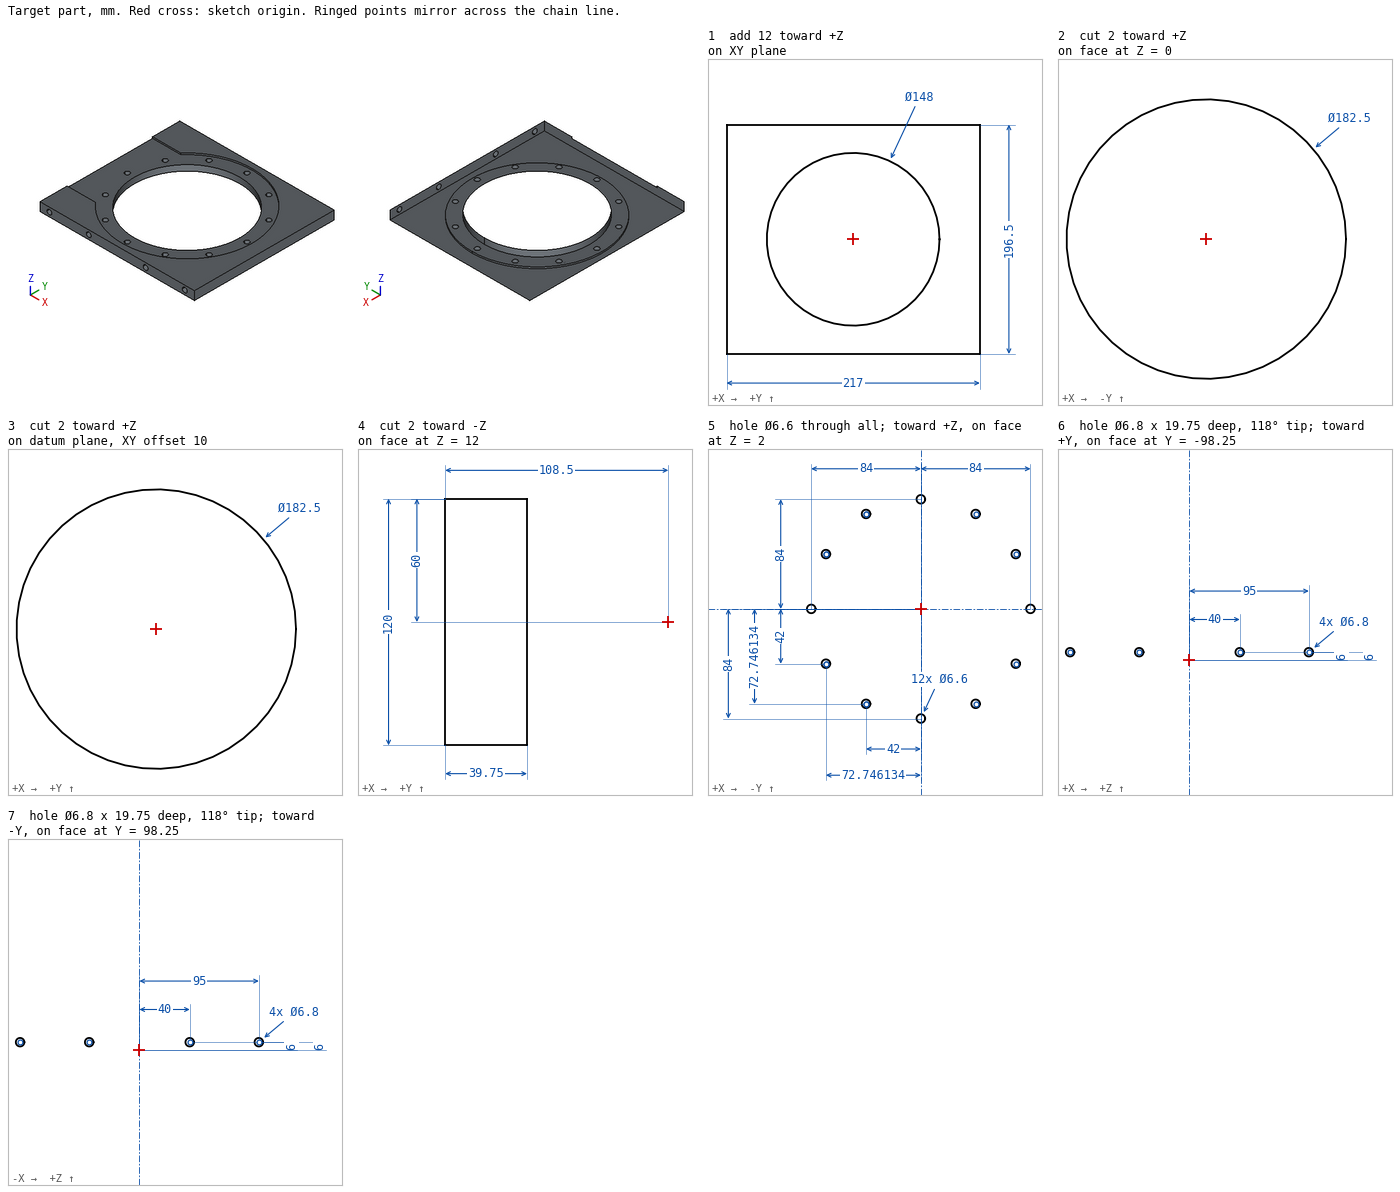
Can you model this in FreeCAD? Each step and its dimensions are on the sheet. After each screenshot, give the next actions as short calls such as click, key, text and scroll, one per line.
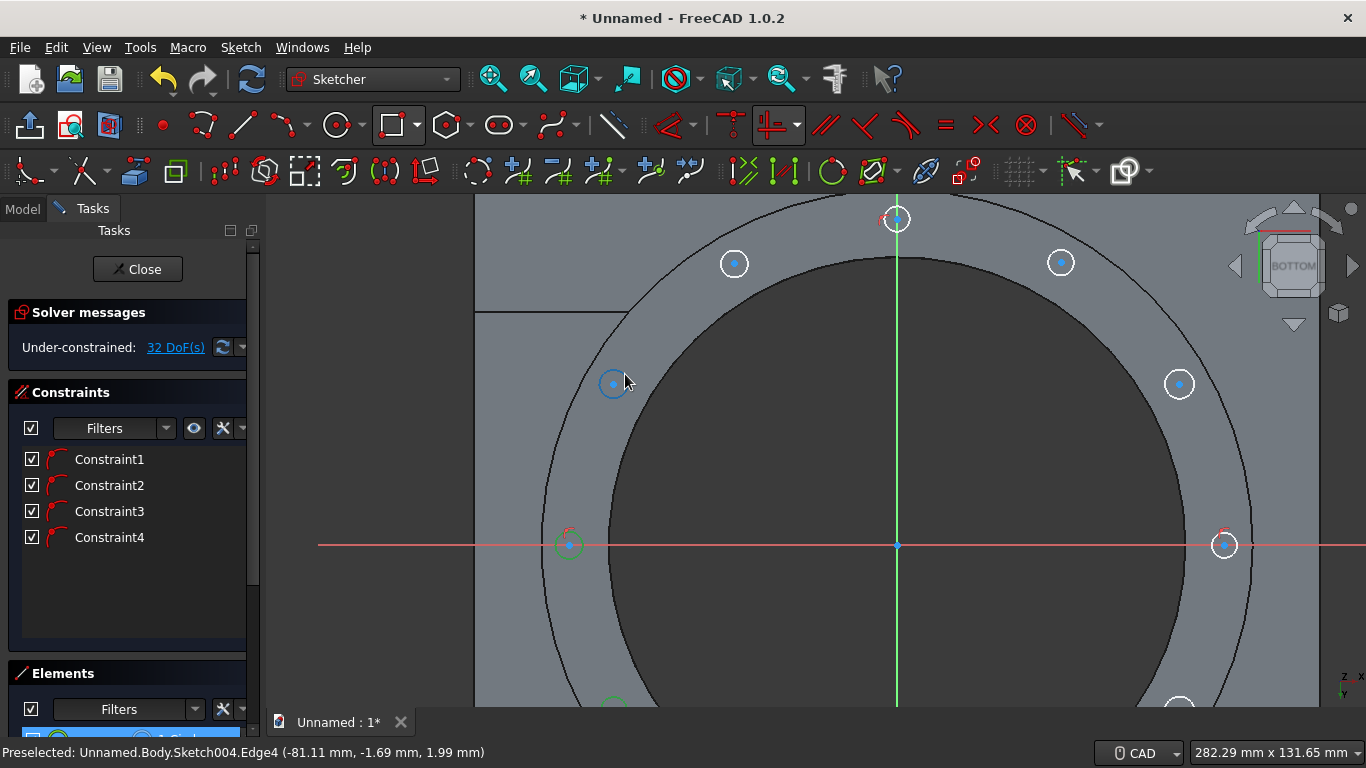
click(624, 374)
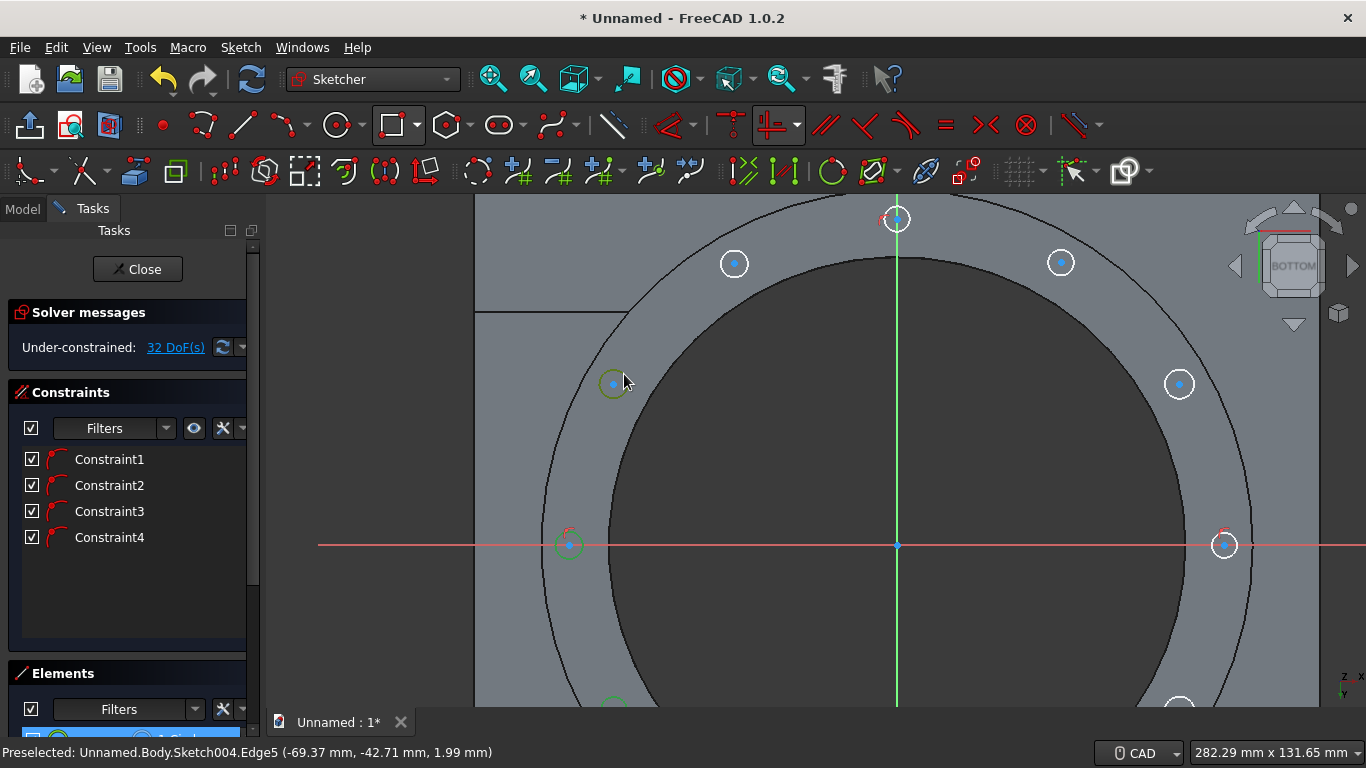
click(744, 254)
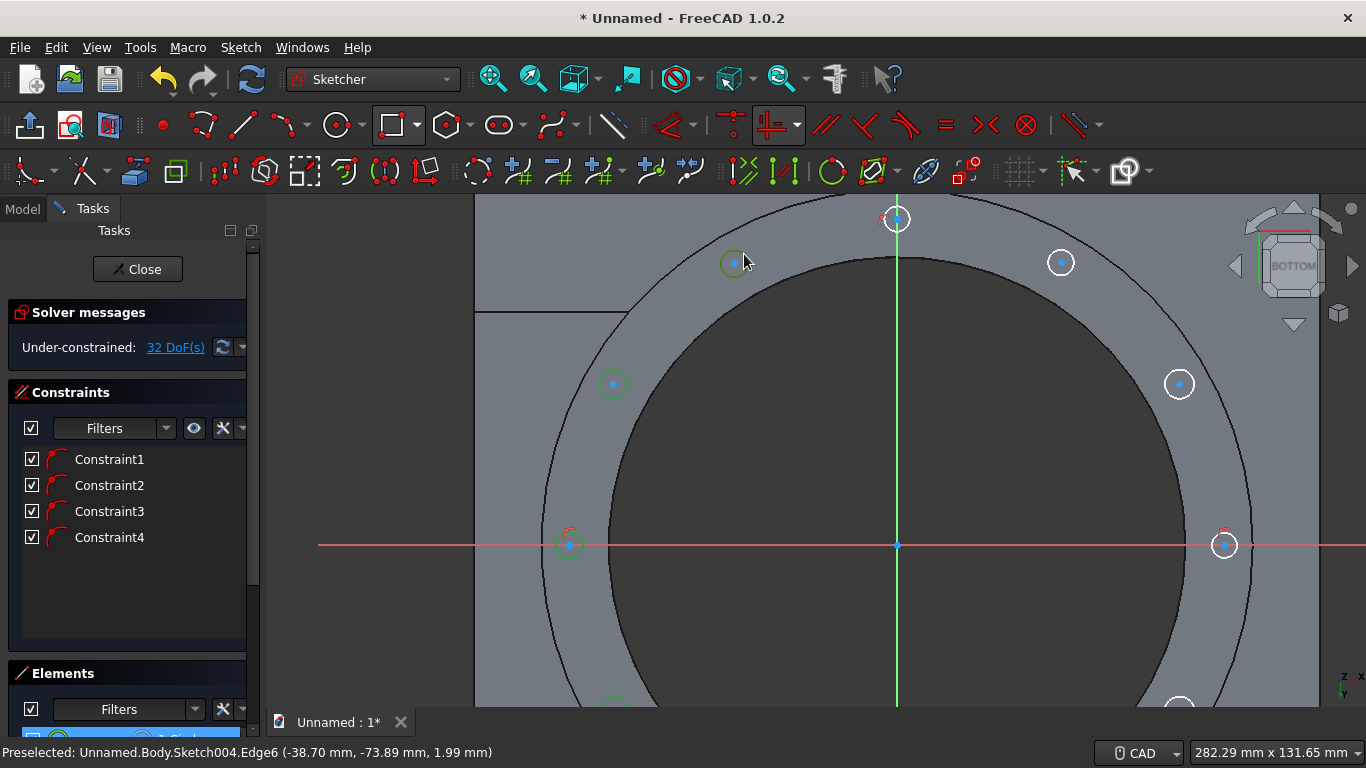
click(897, 232)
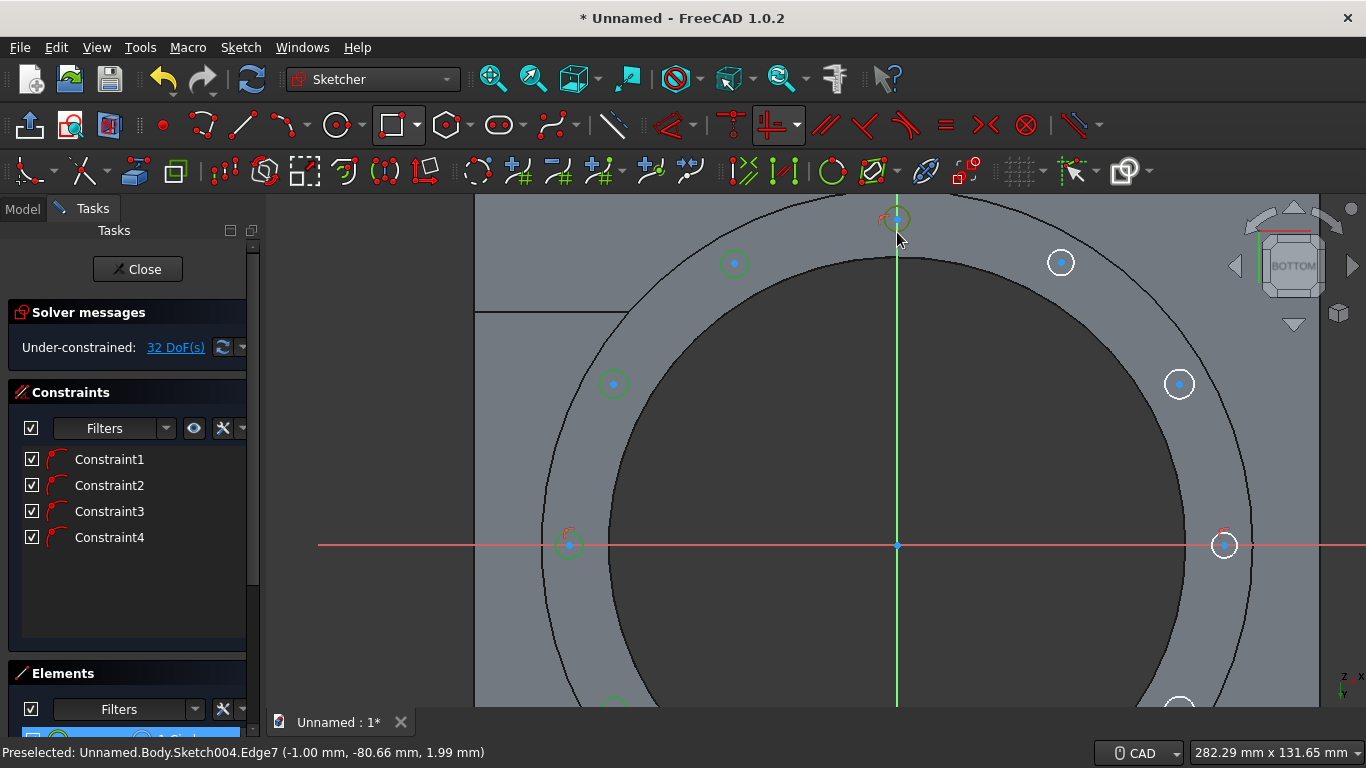
click(1070, 254)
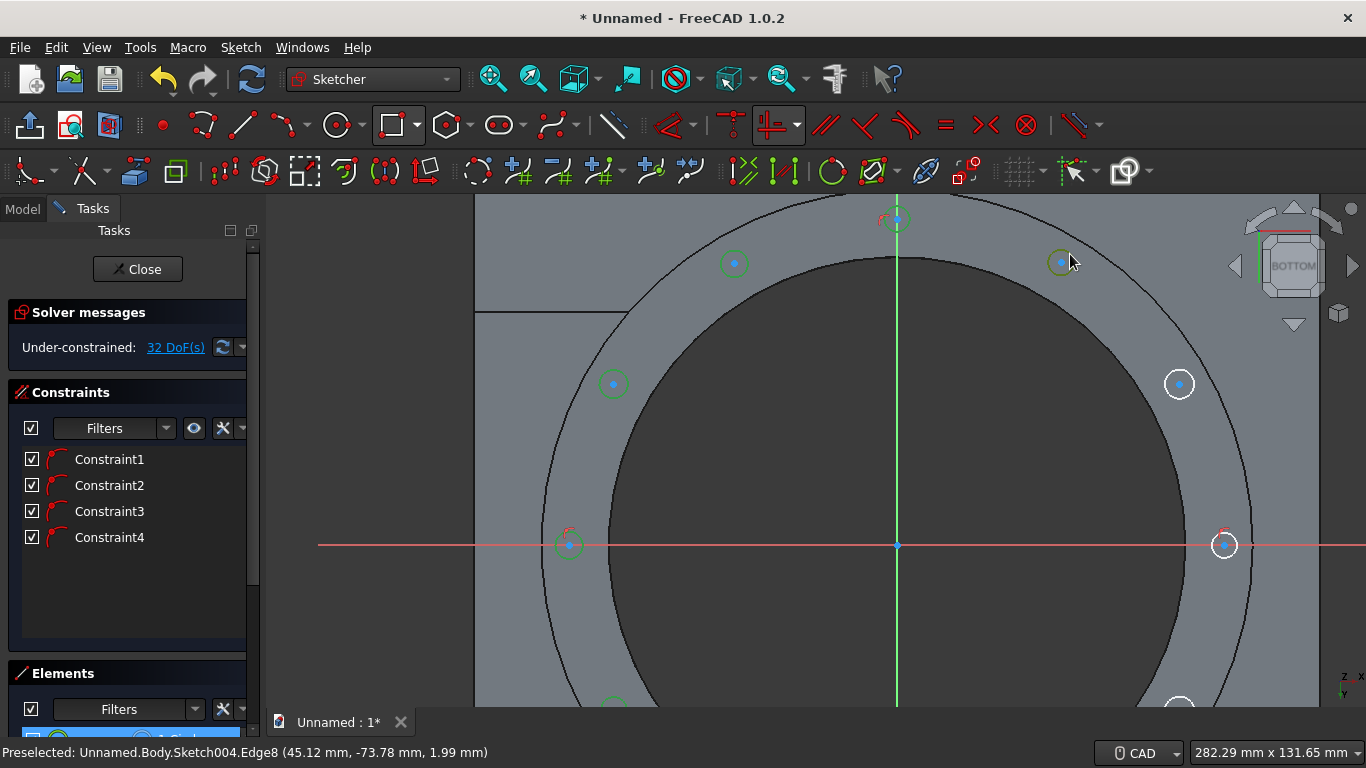
click(1190, 374)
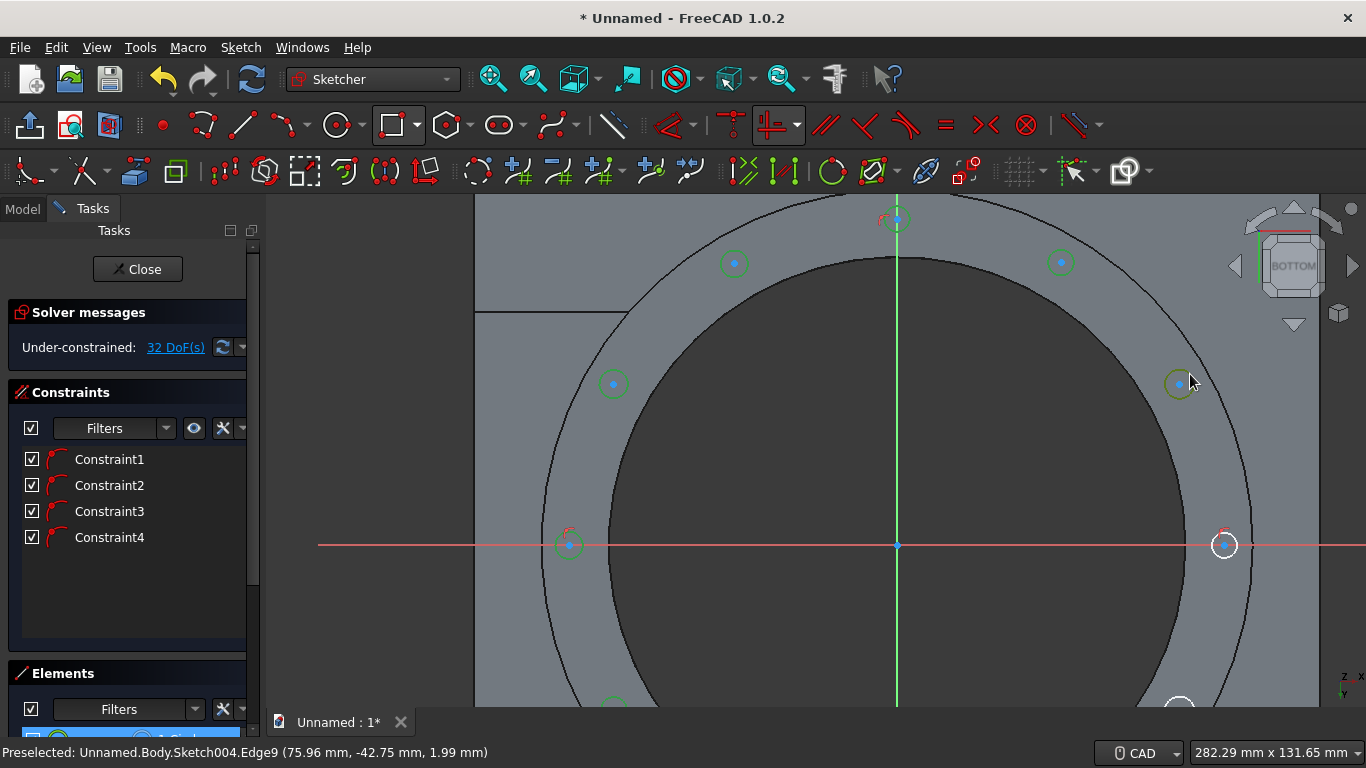
scroll(625, 373, down, 4)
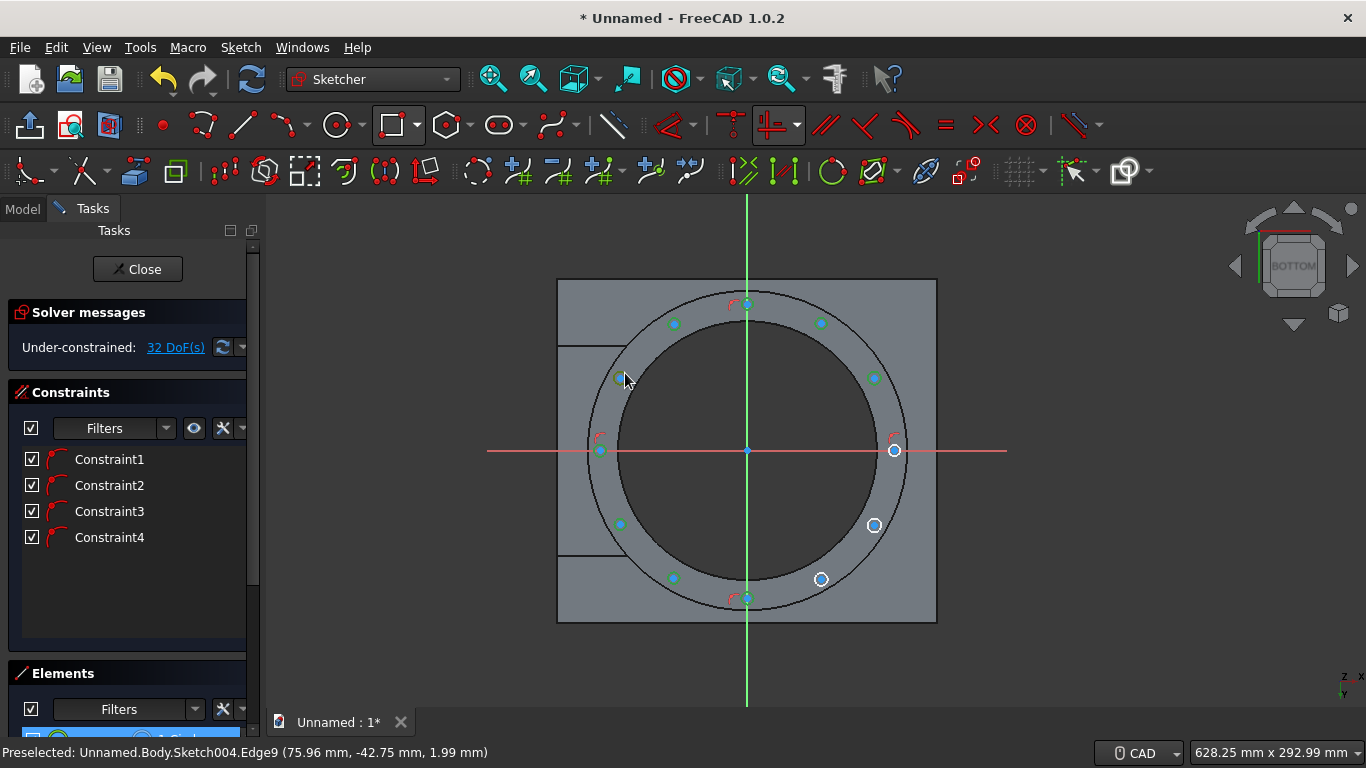
scroll(895, 445, up, 5)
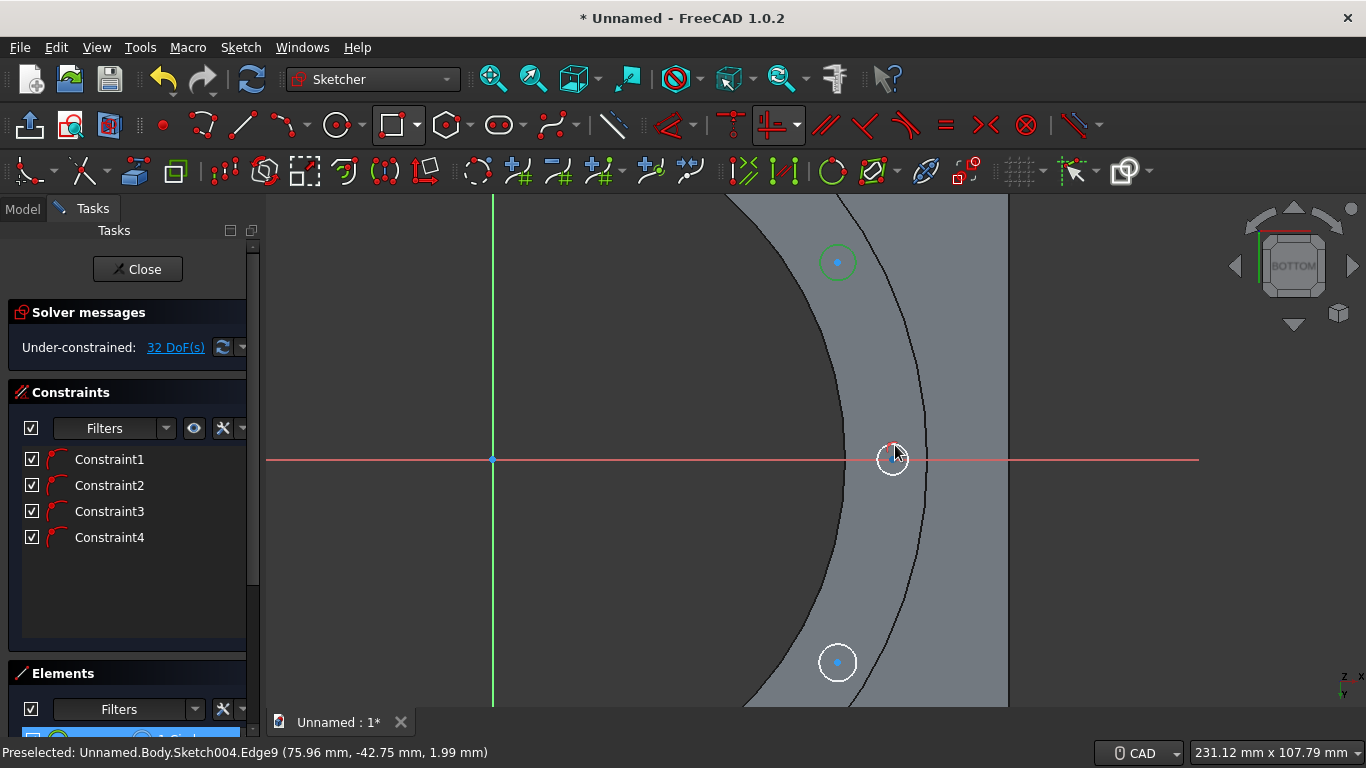
click(877, 459)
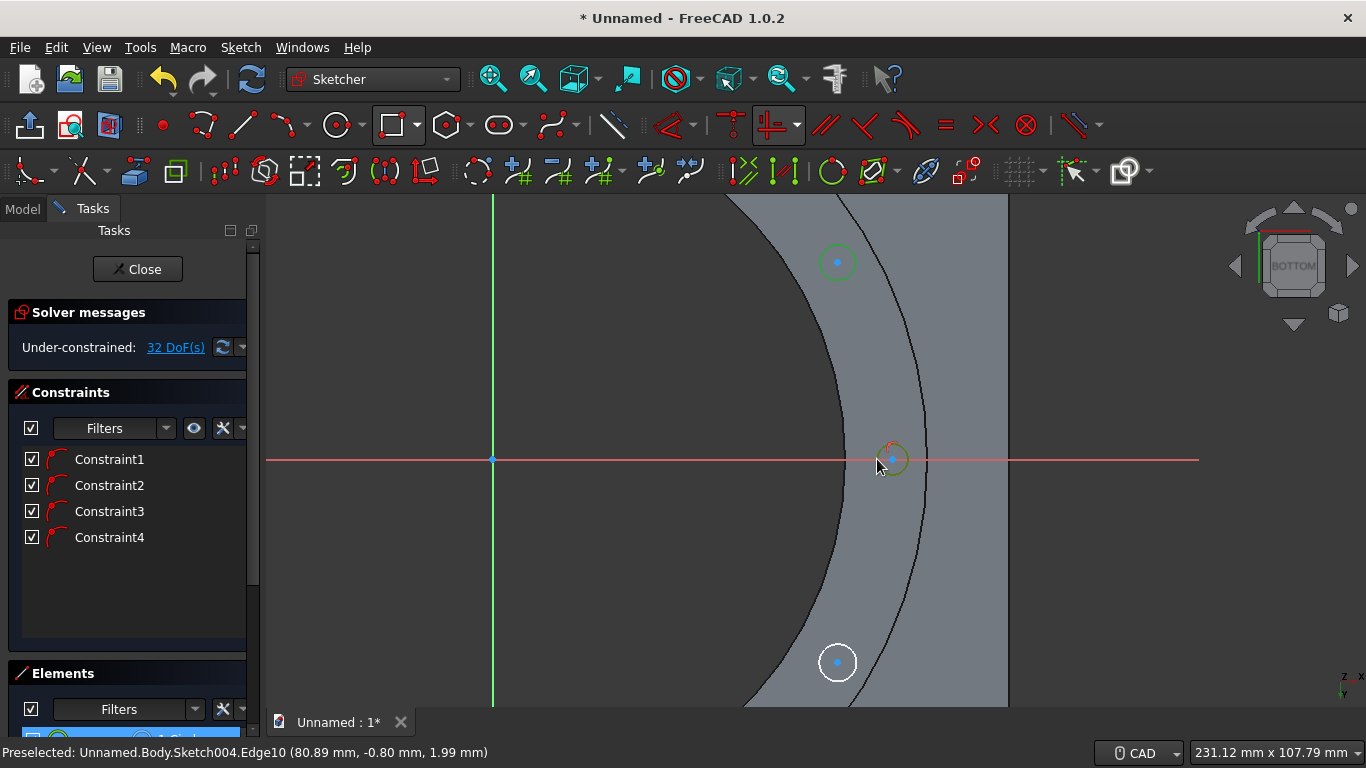
click(851, 650)